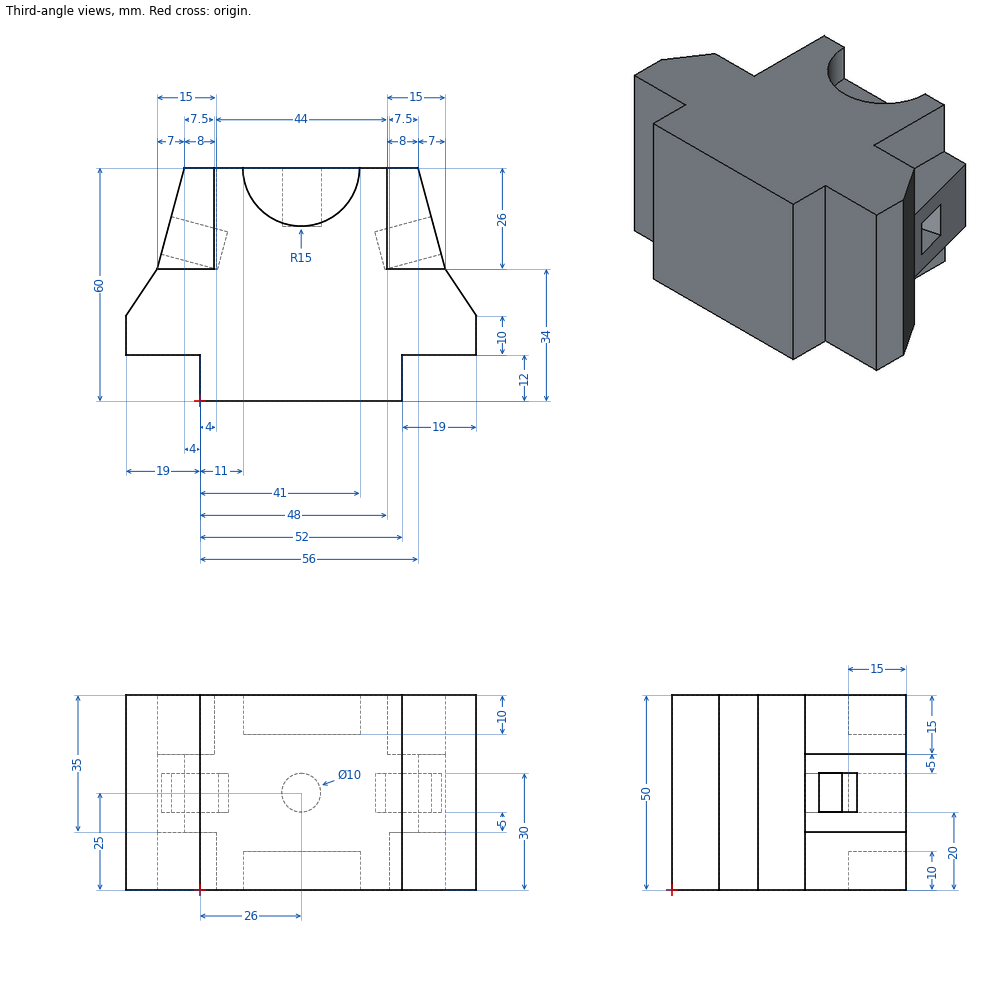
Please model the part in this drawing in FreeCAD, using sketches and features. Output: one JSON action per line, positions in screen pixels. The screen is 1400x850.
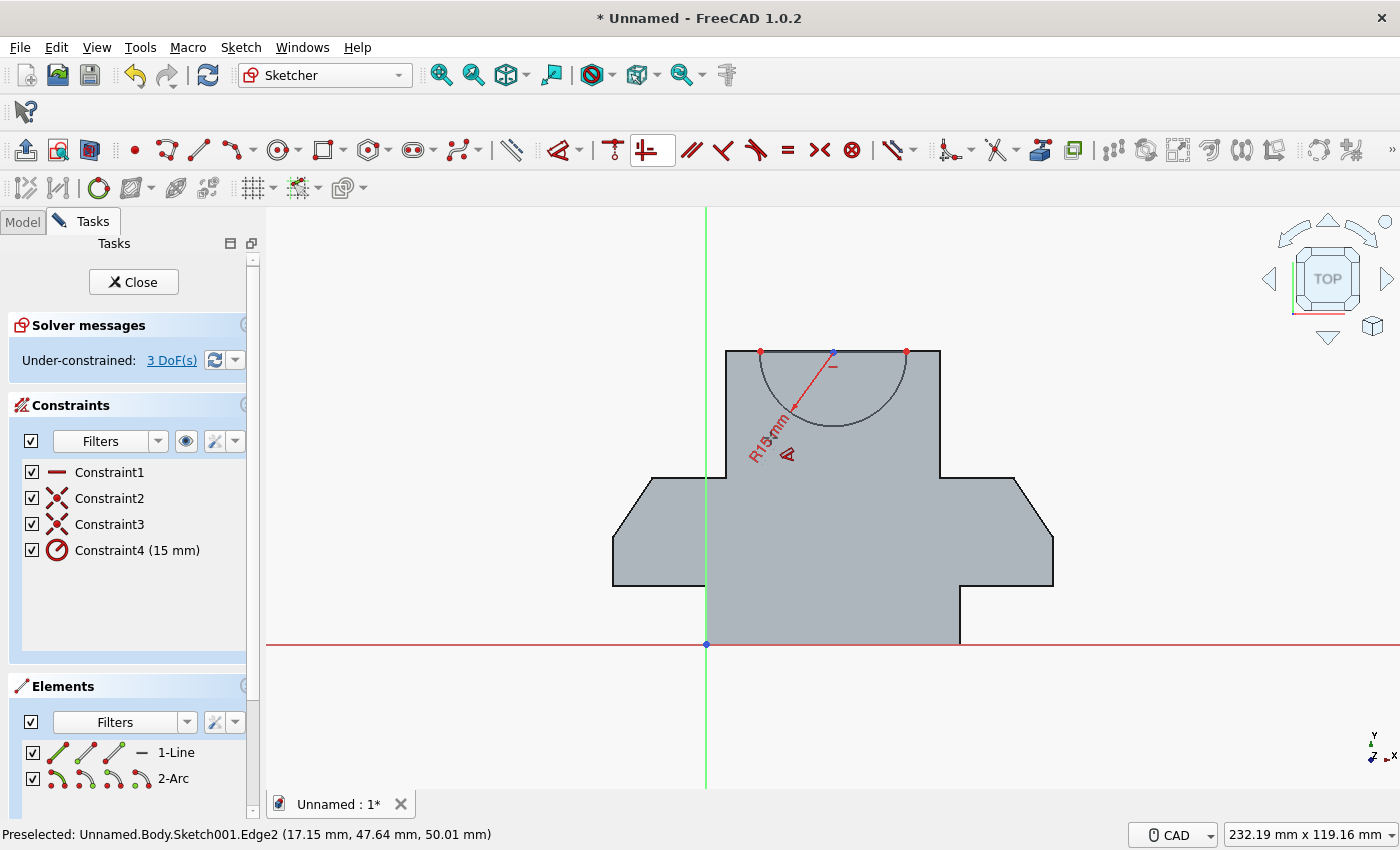
{"action": "left_click", "coordinate": [907, 352]}
{"action": "left_click", "coordinate": [806, 679]}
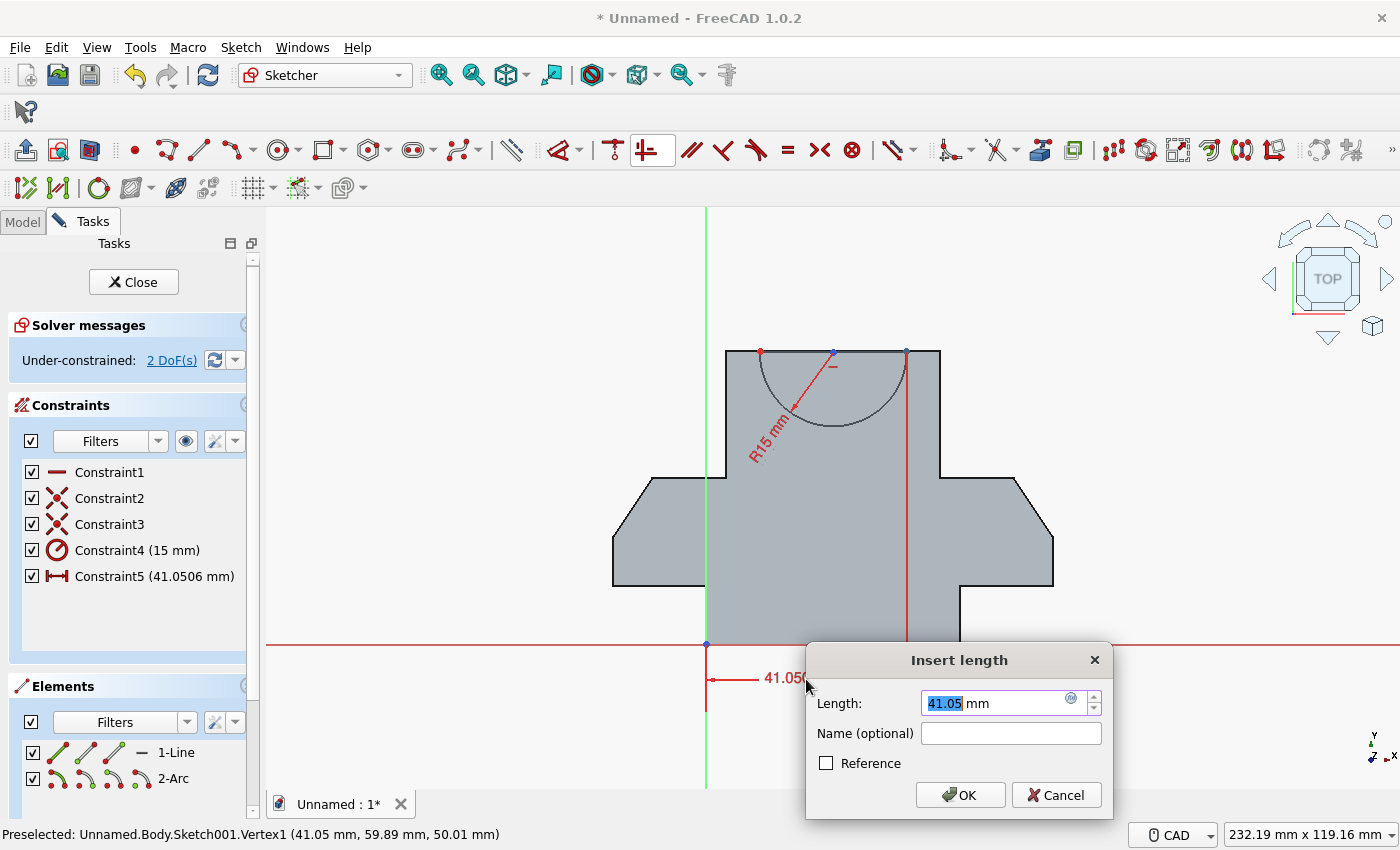
{"action": "type", "text": "41"}
{"action": "key", "text": "Return"}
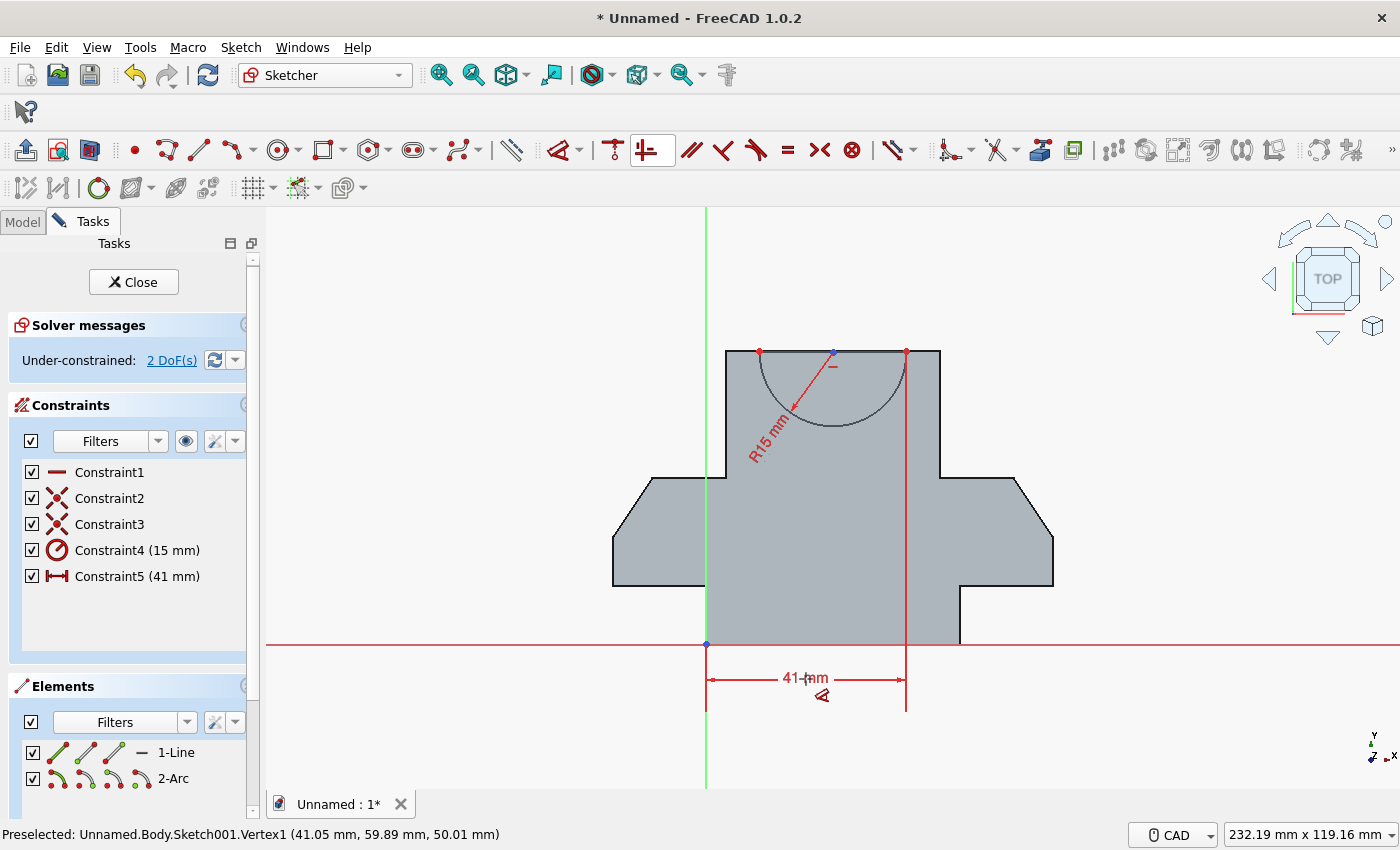
{"action": "left_click", "coordinate": [906, 352]}
{"action": "left_click", "coordinate": [940, 498]}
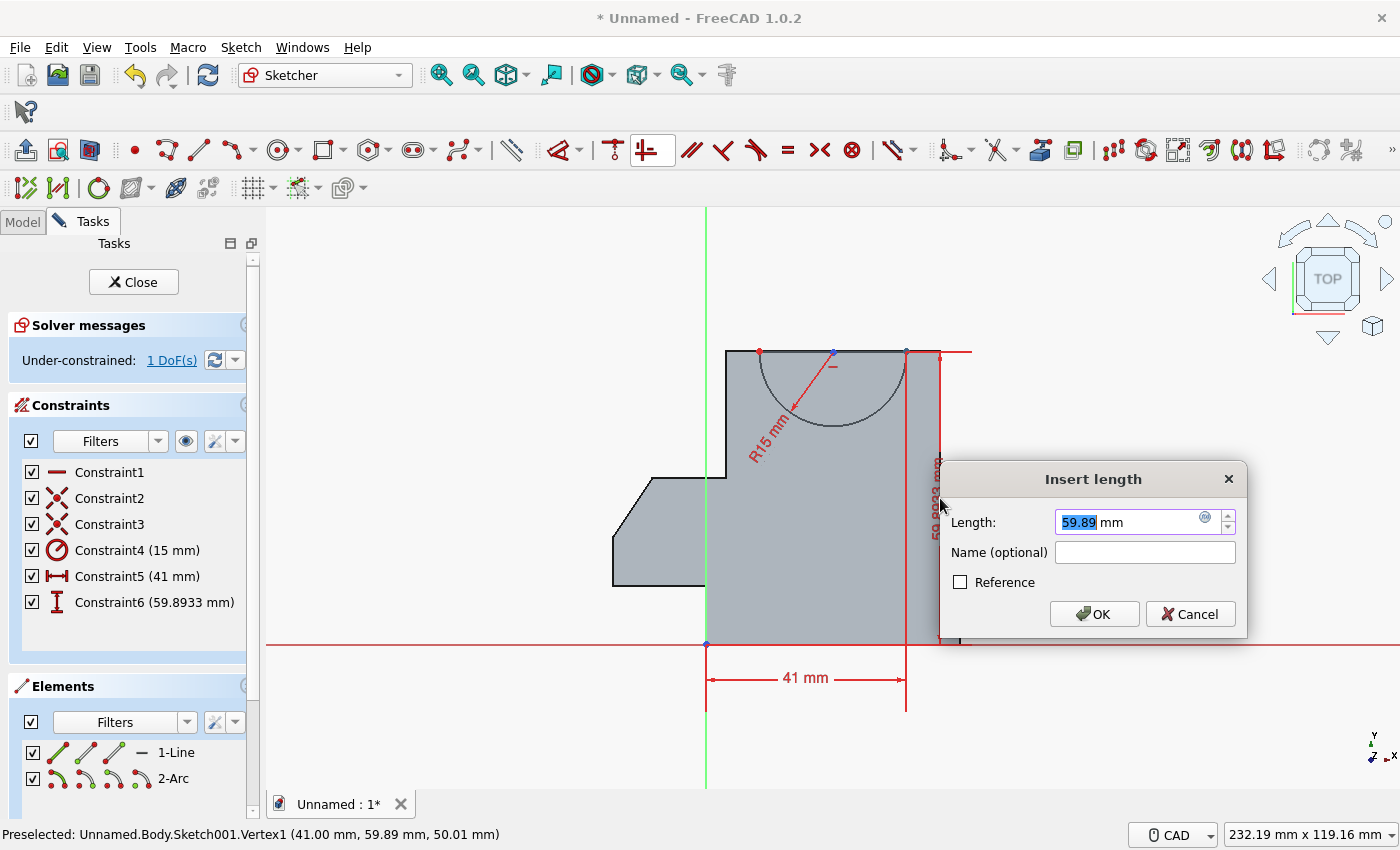
{"action": "type", "text": "60"}
{"action": "key", "text": "Return"}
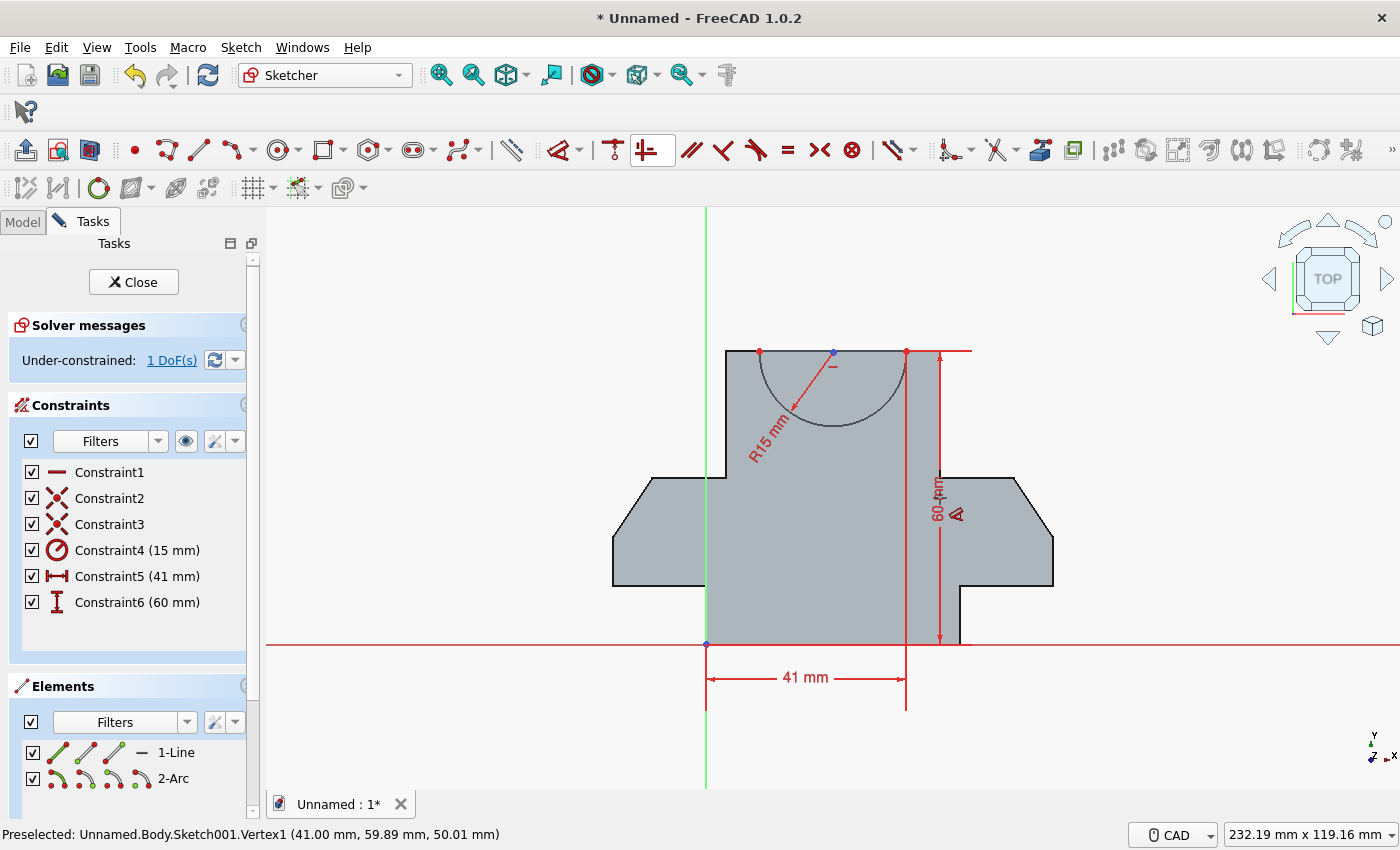
{"action": "left_click", "coordinate": [833, 353]}
{"action": "left_click", "coordinate": [672, 499]}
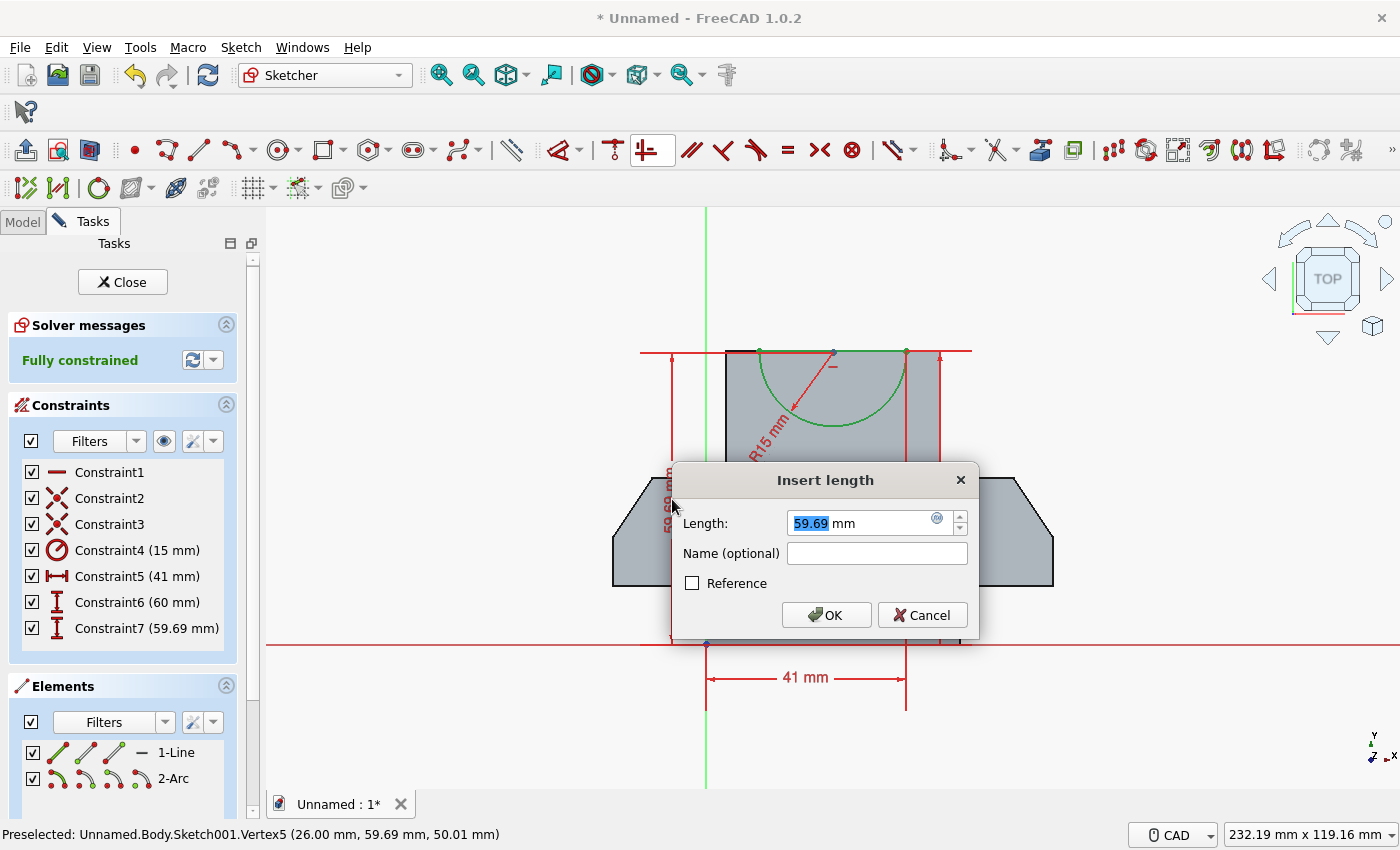
{"action": "type", "text": "60"}
{"action": "key", "text": "Return"}
{"action": "key", "text": "Escape"}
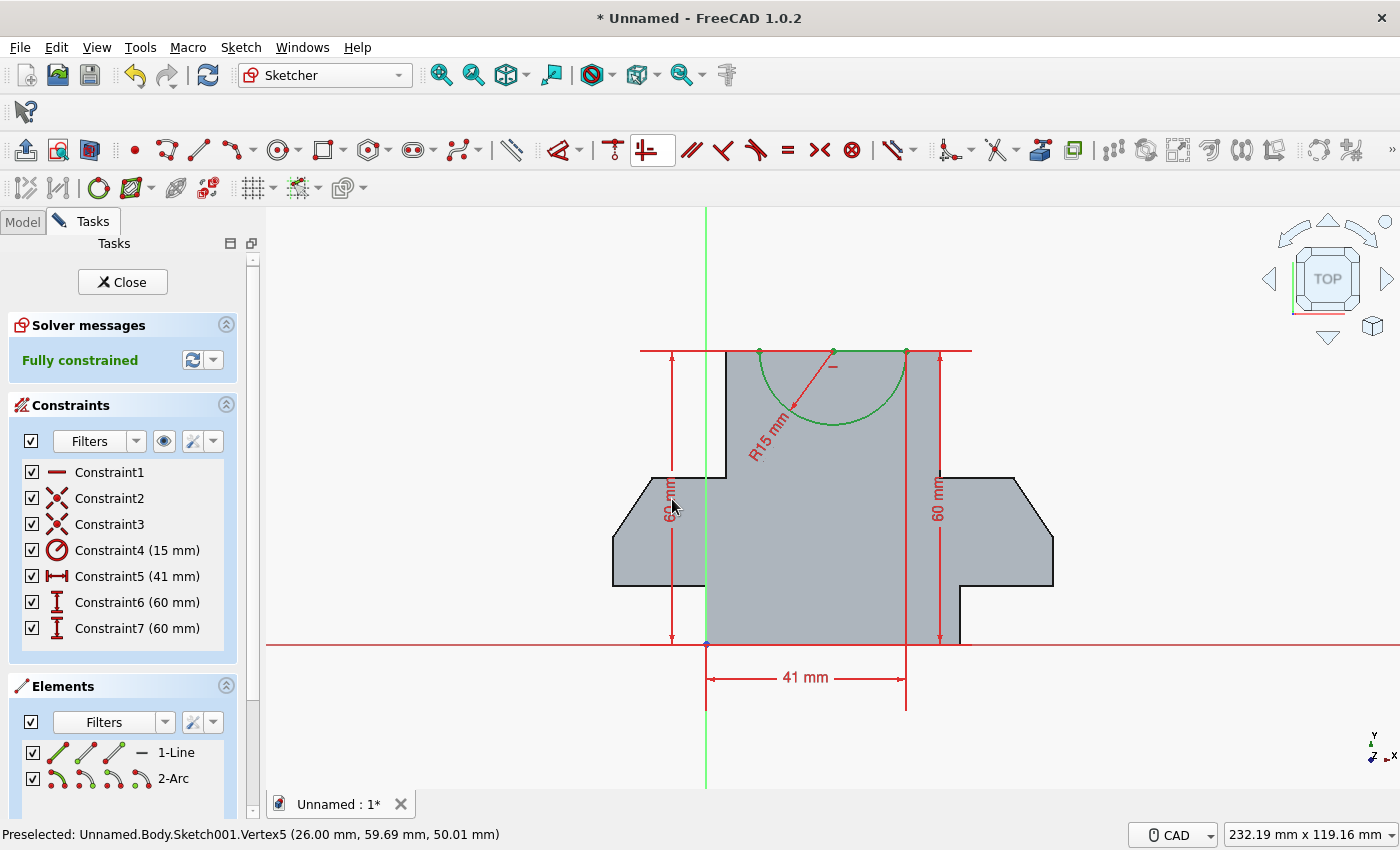
{"action": "left_click", "coordinate": [123, 282]}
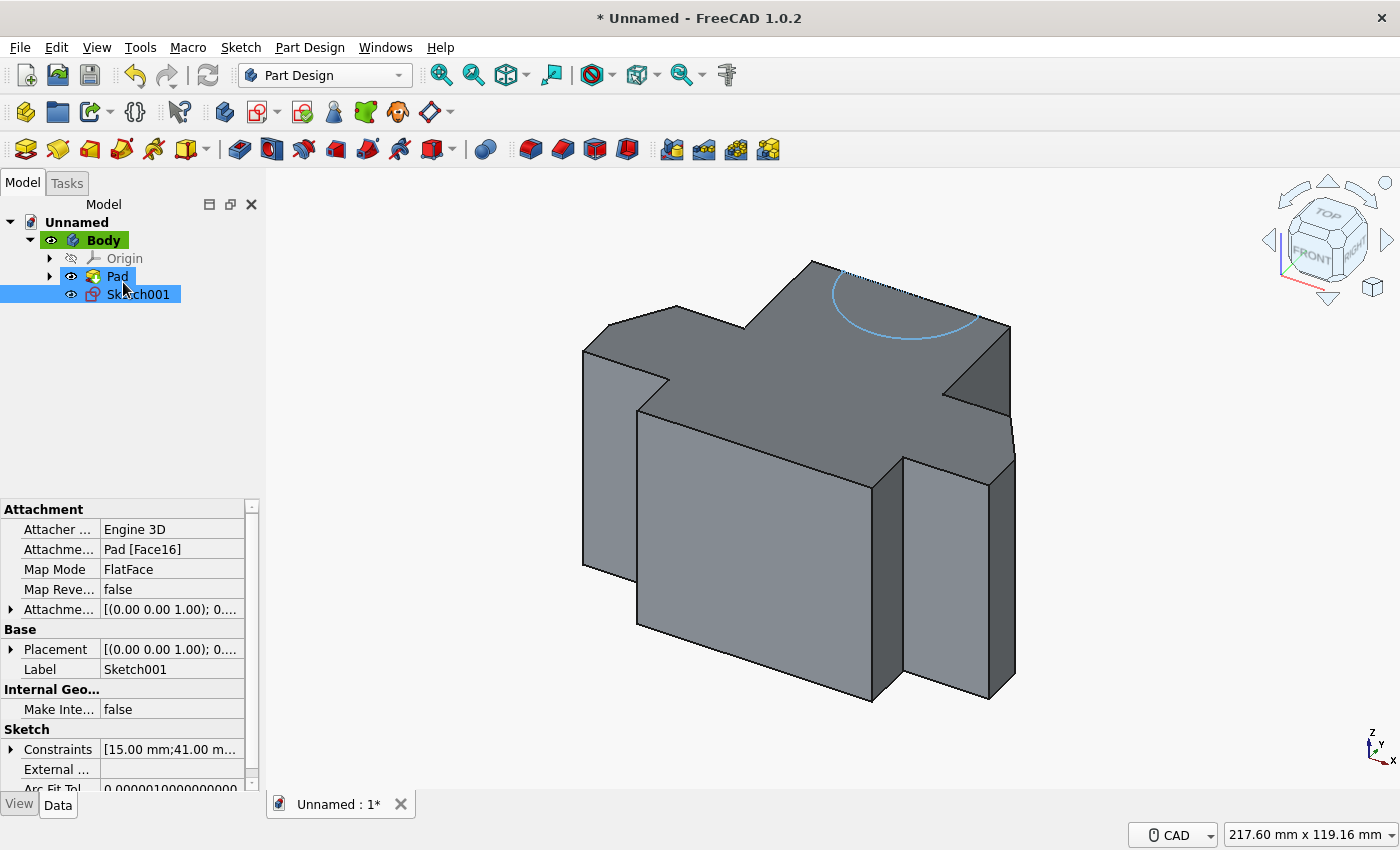
{"action": "left_click", "coordinate": [240, 150]}